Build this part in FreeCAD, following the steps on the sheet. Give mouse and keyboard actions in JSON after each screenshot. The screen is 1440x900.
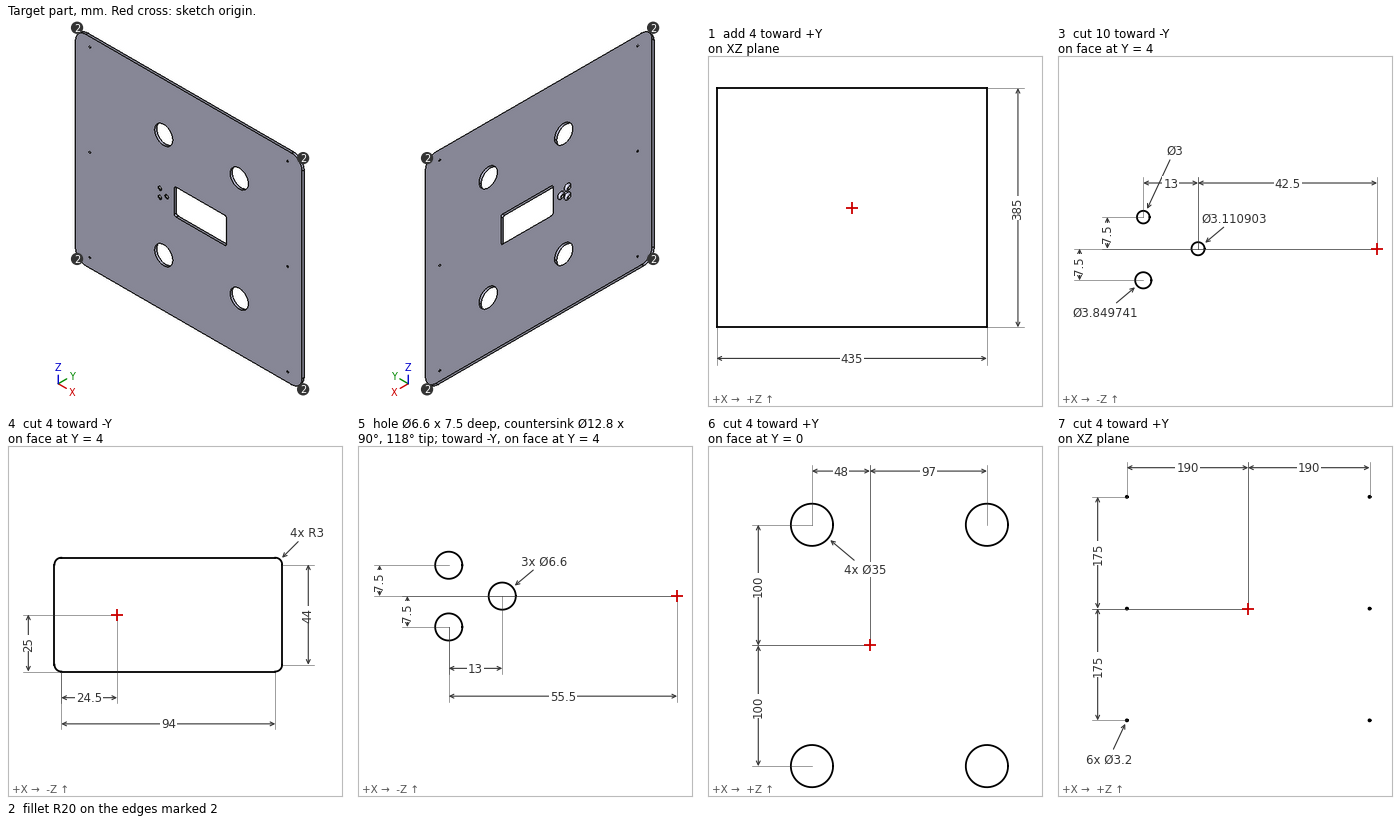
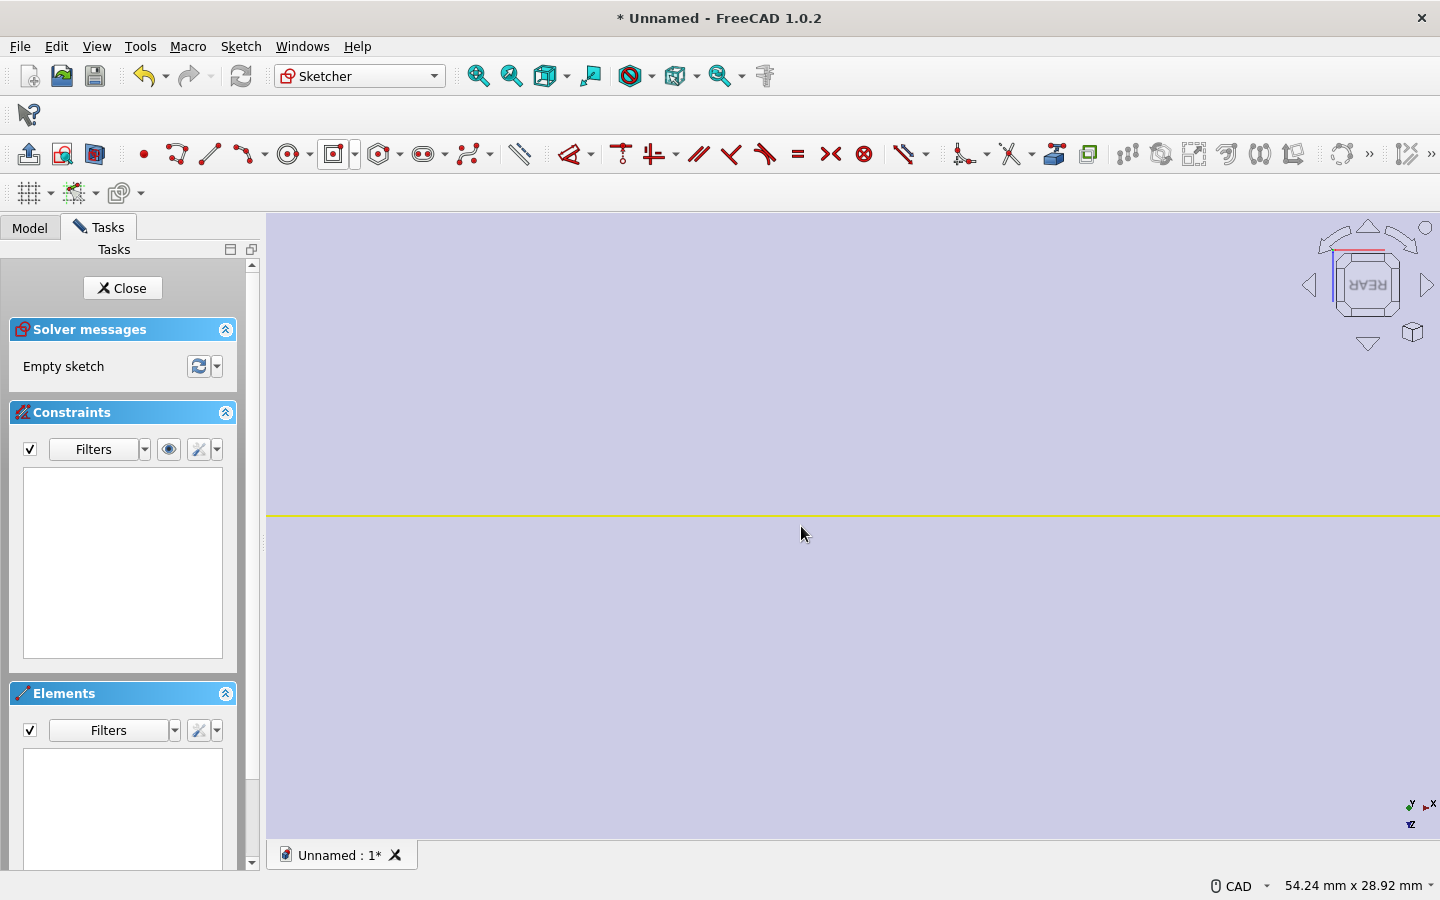
{"action": "left_click", "coordinate": [288, 154]}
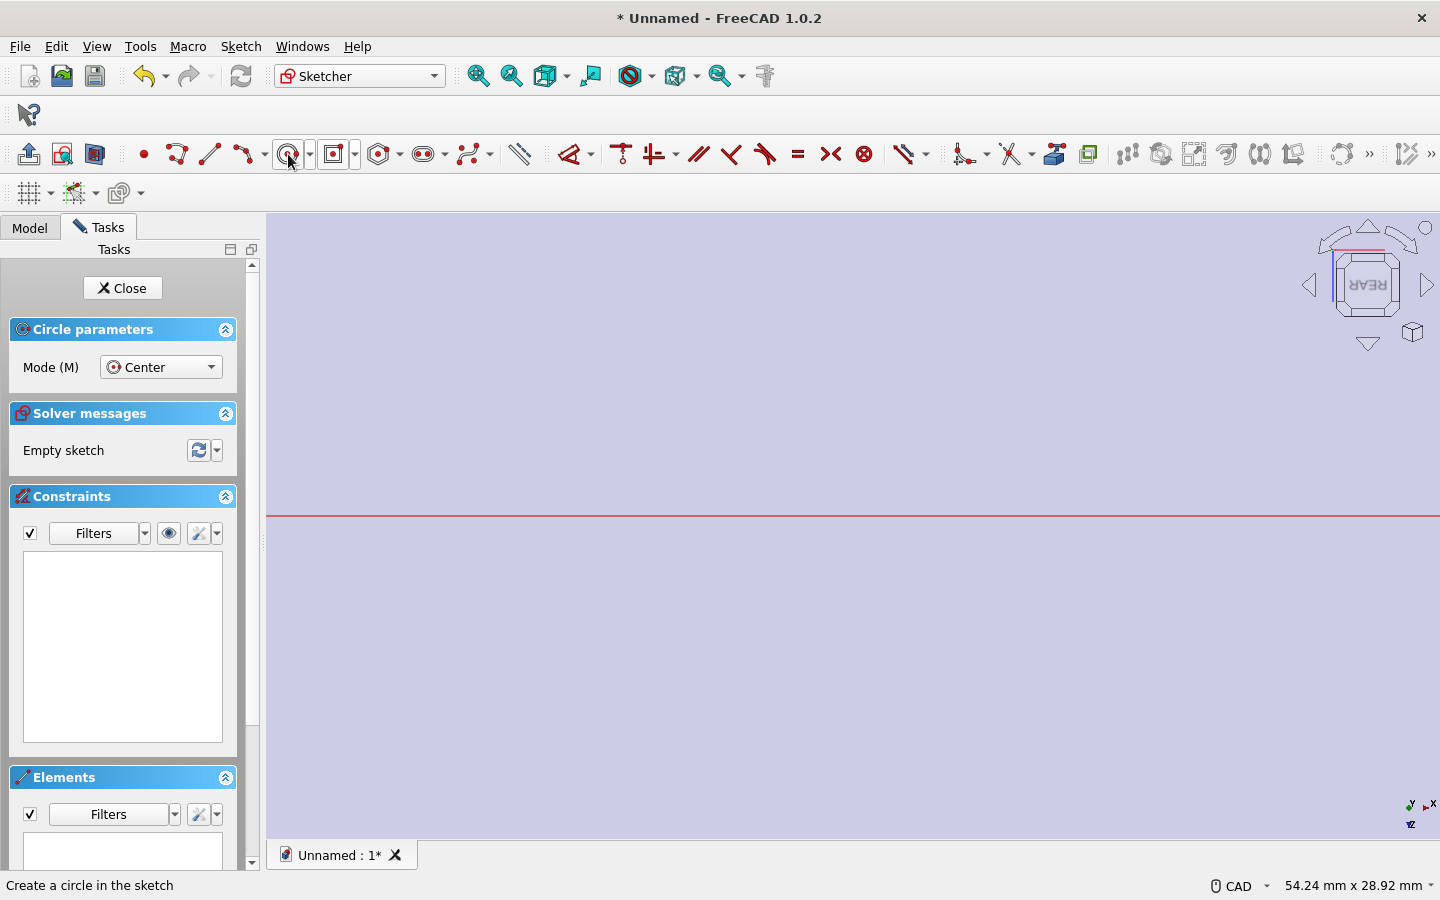
{"action": "left_click", "coordinate": [917, 516]}
{"action": "left_click", "coordinate": [941, 493]}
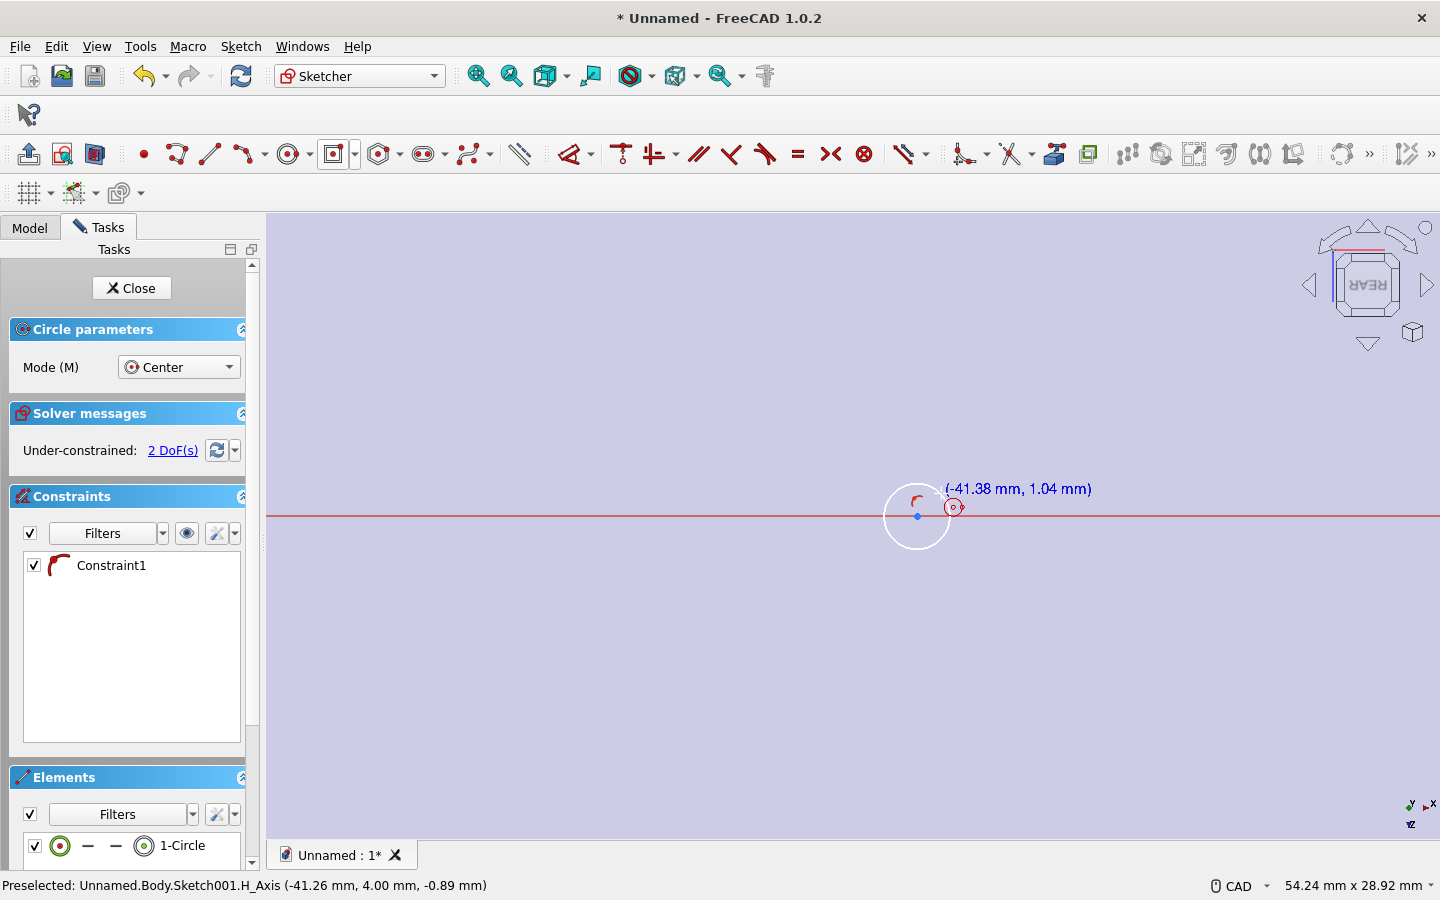
{"action": "left_click", "coordinate": [635, 354]}
{"action": "left_click", "coordinate": [658, 331]}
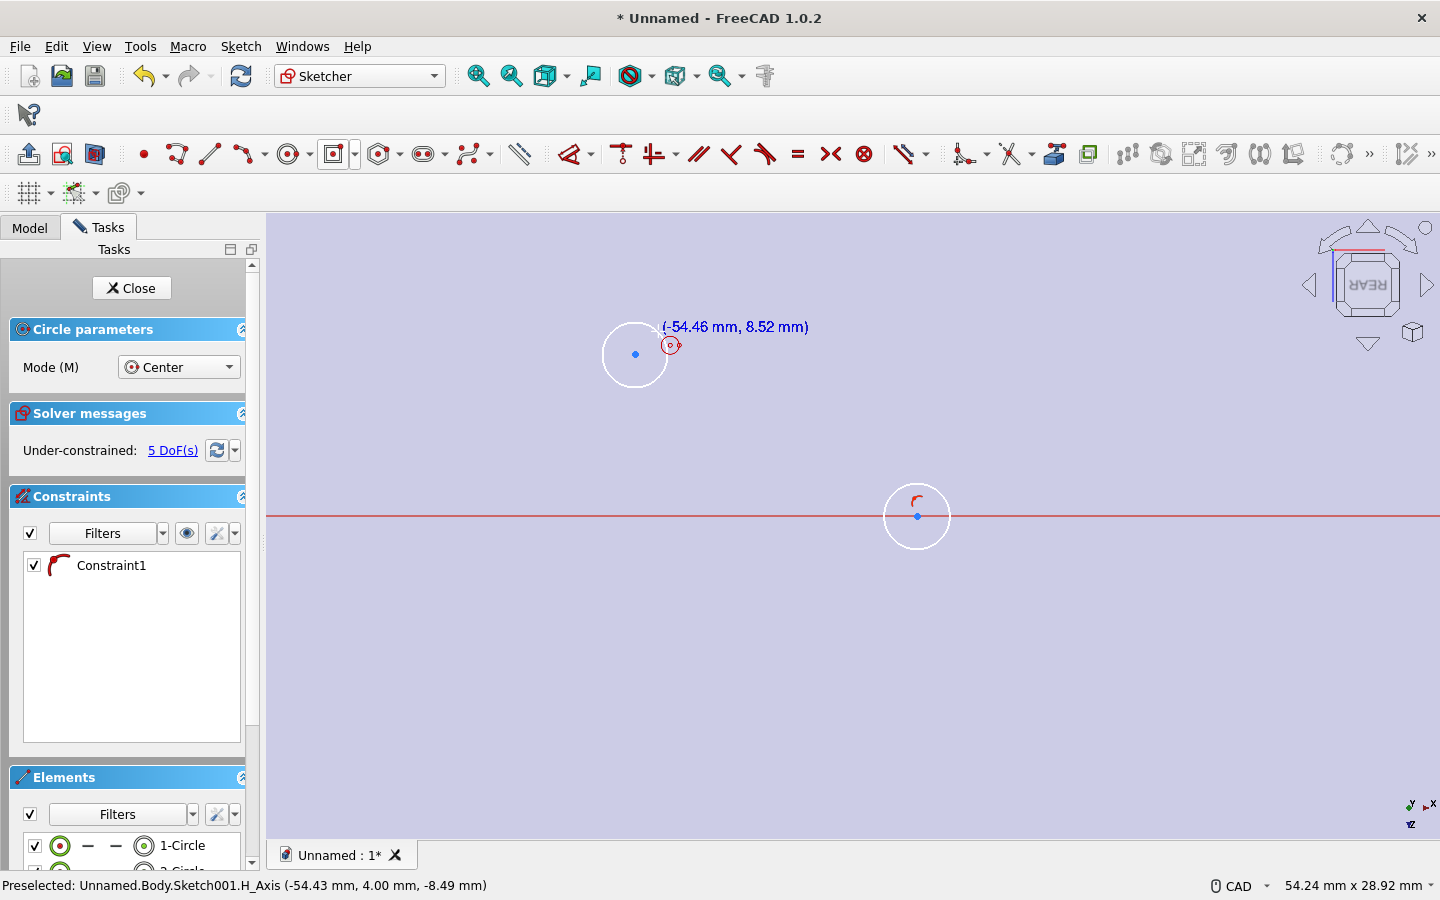
{"action": "left_click", "coordinate": [635, 679]}
{"action": "left_click", "coordinate": [665, 649]}
{"action": "key", "text": "Escape"}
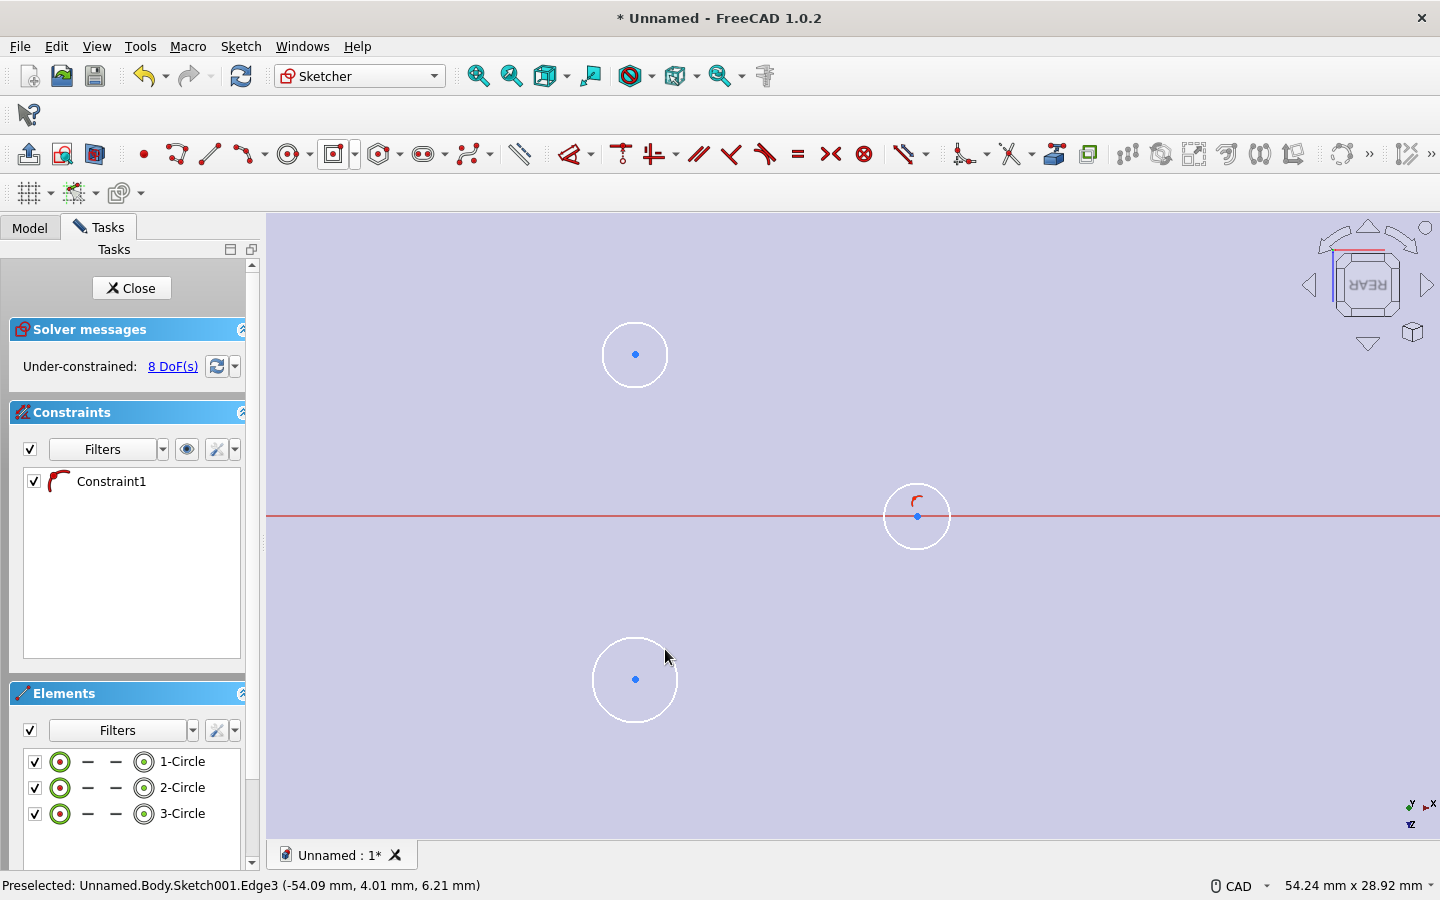
{"action": "left_click", "coordinate": [635, 355]}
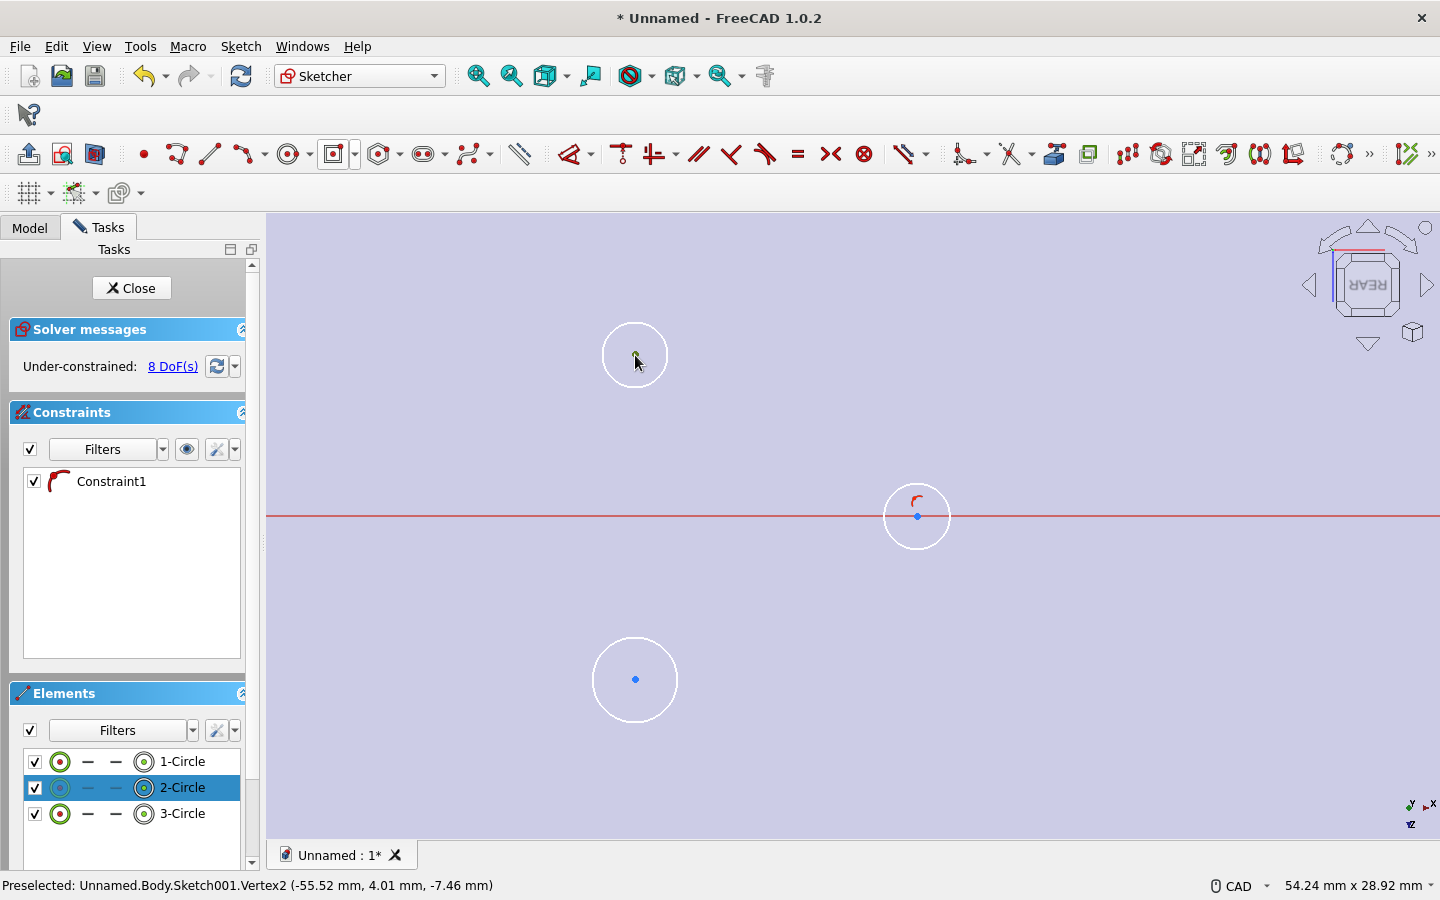
{"action": "left_click", "coordinate": [635, 680]}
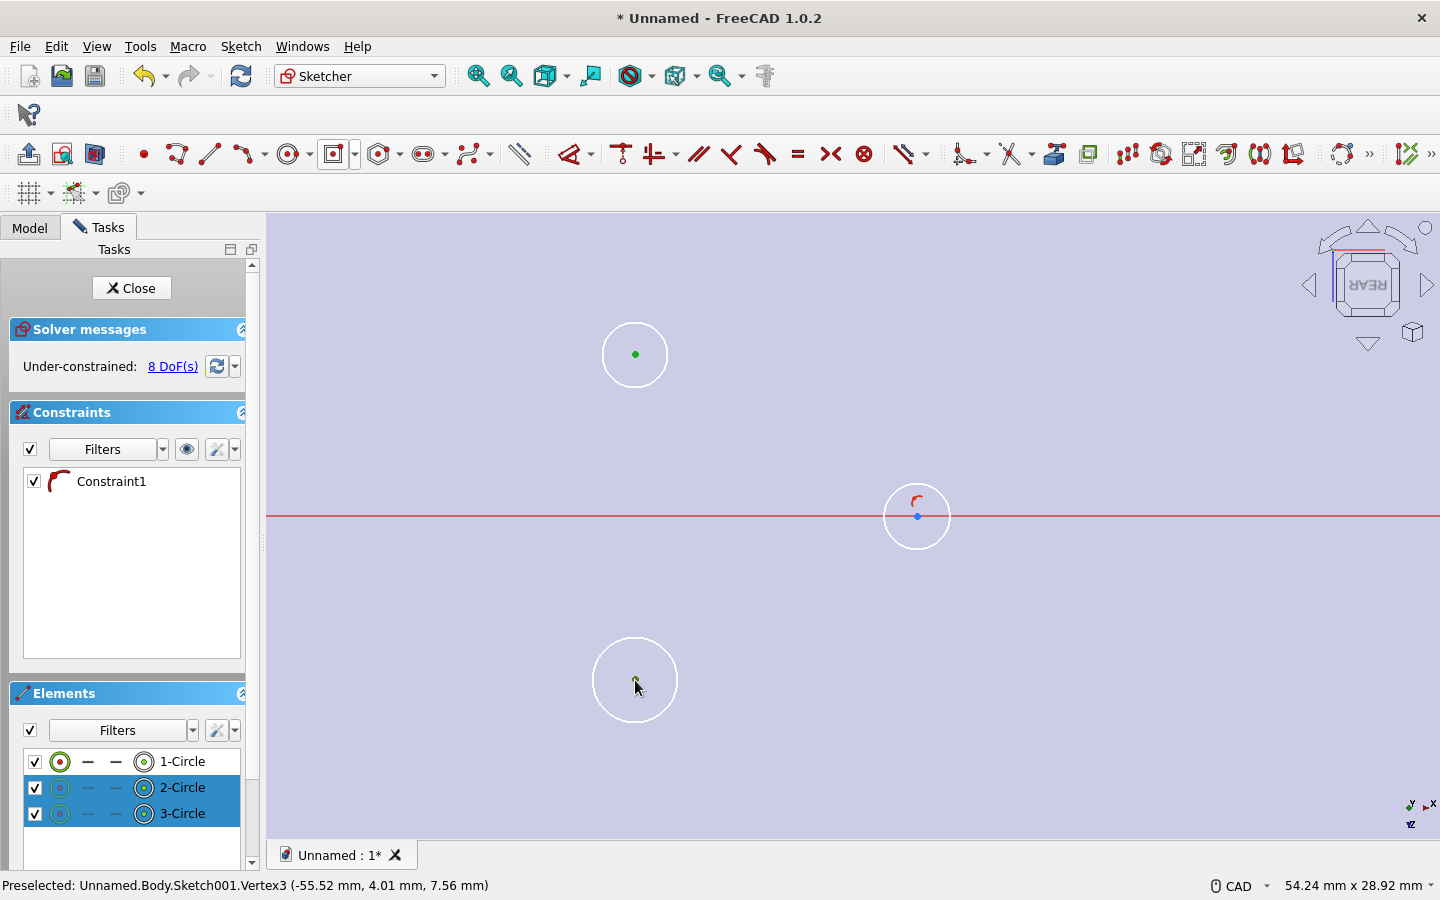
{"action": "key", "text": "v"}